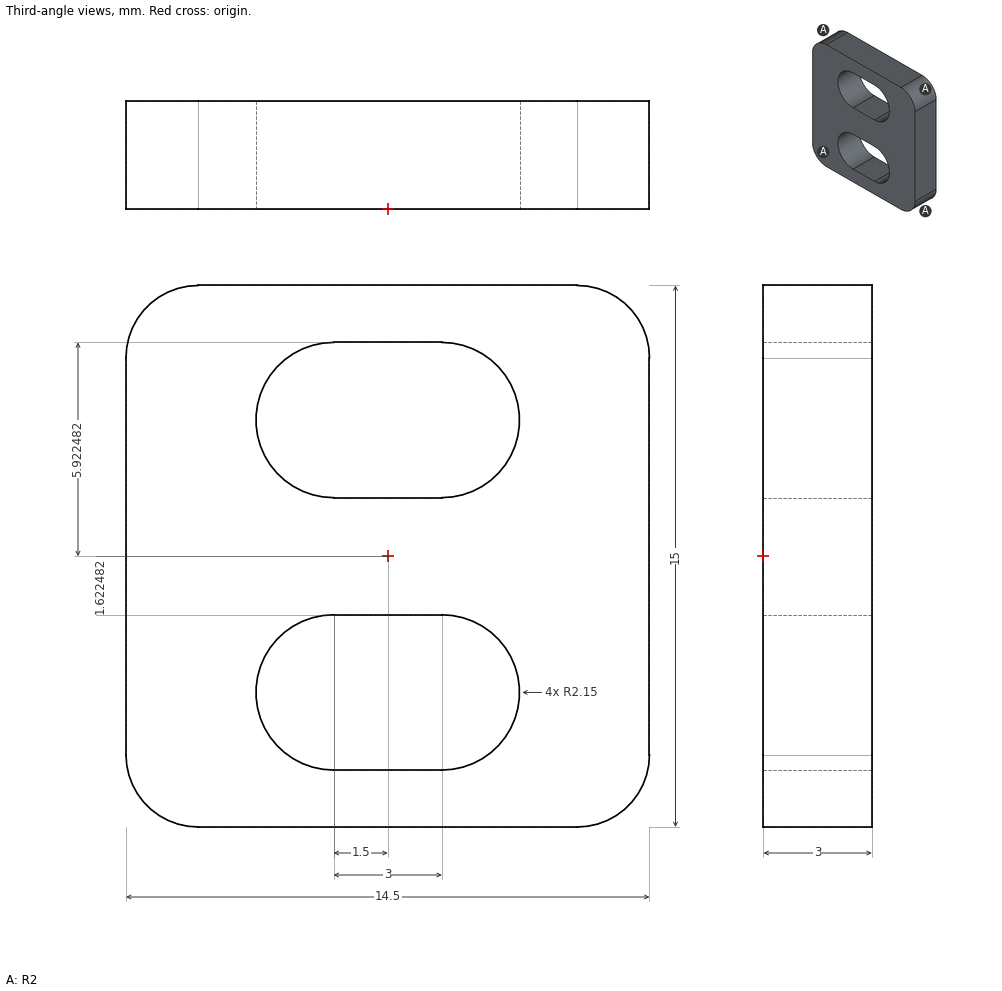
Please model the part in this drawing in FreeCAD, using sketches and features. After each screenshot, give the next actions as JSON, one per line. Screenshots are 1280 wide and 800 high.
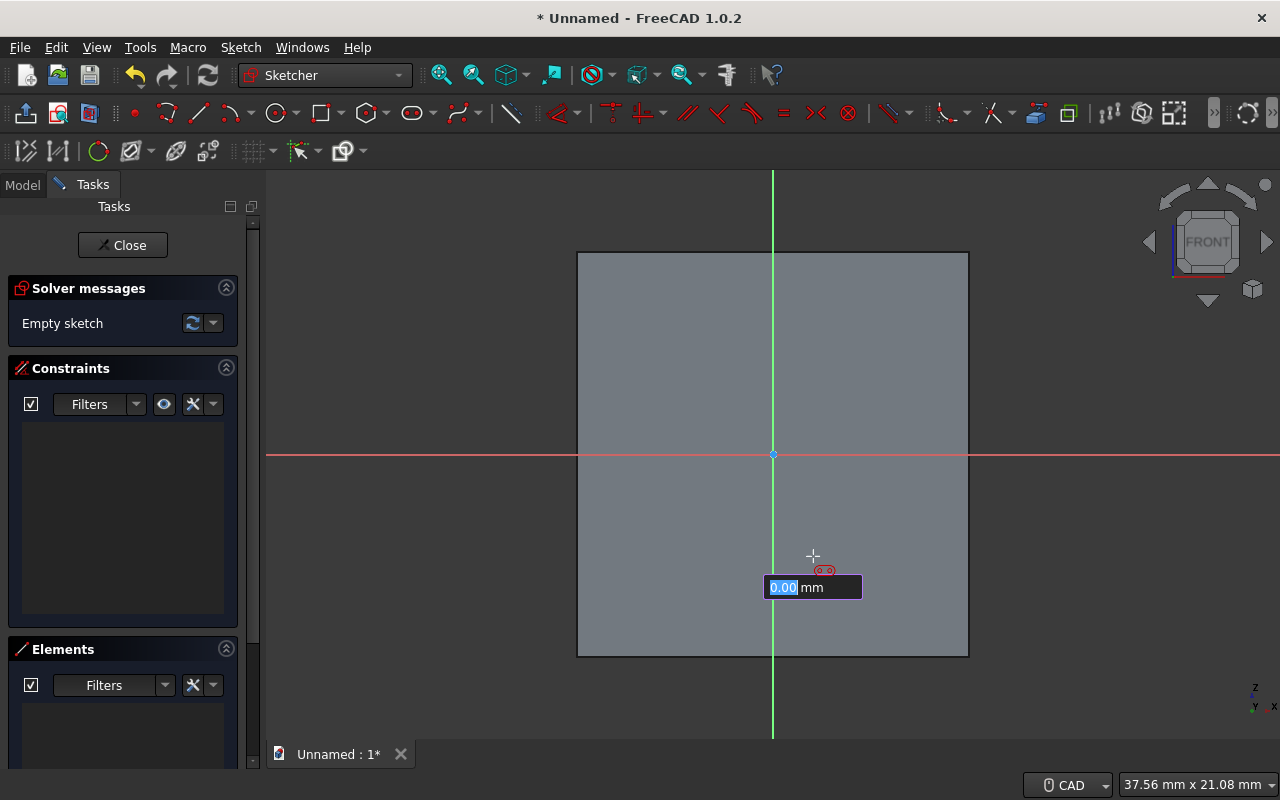
{"action": "scroll", "coordinate": [761, 614], "scroll_direction": "up", "scroll_amount": 2}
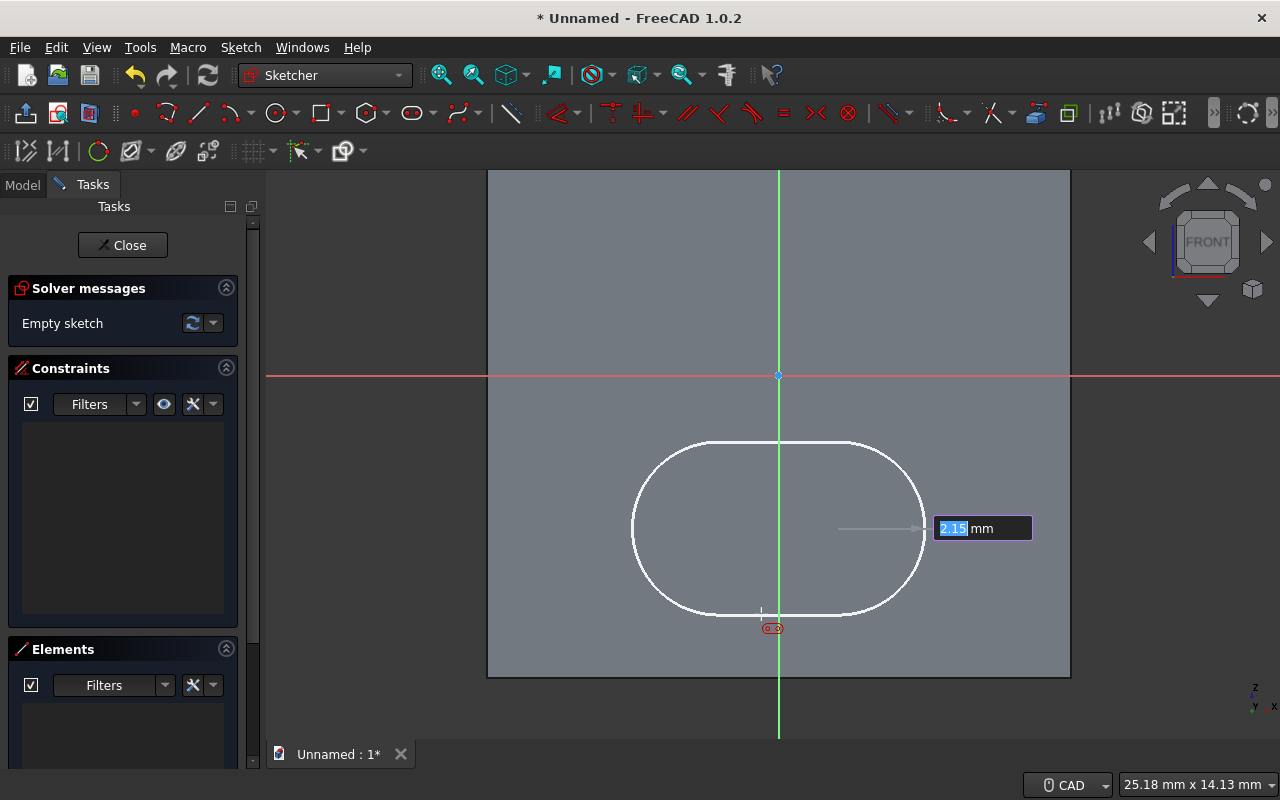
{"action": "left_click", "coordinate": [761, 614]}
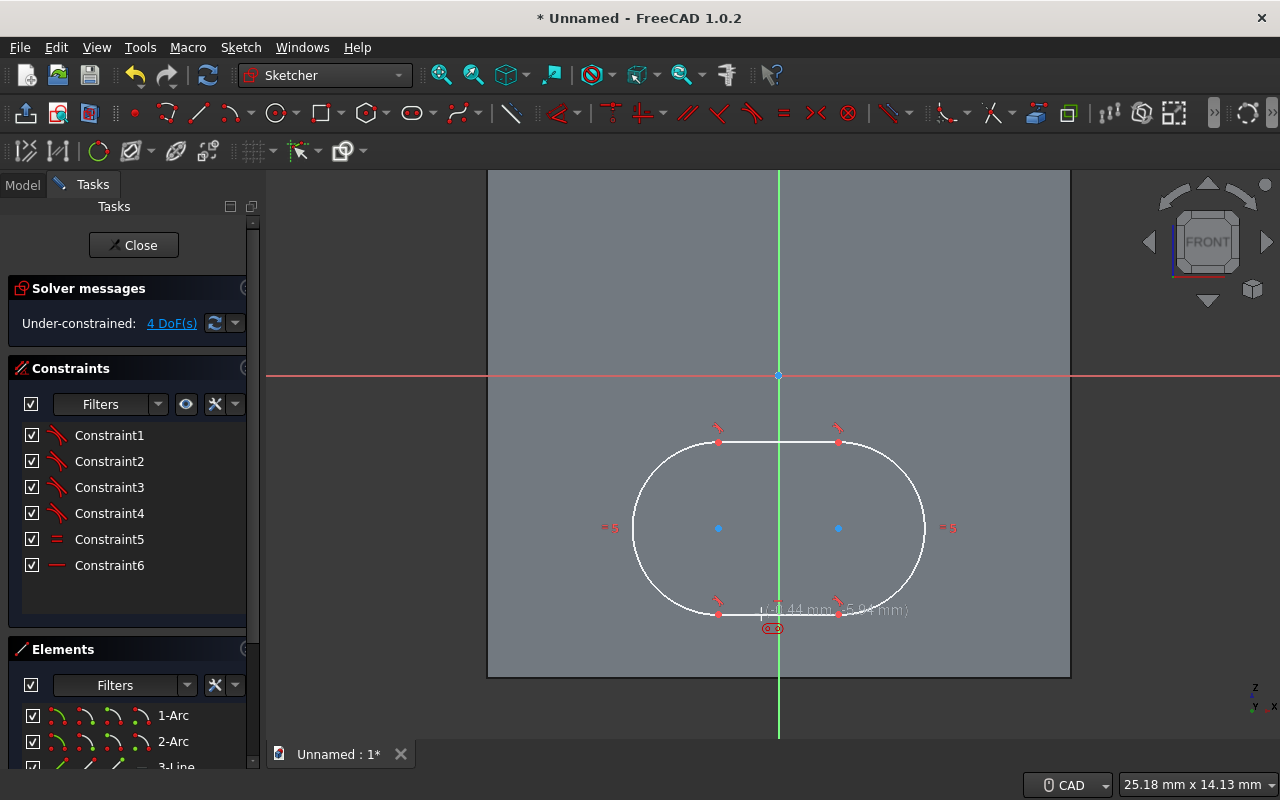
{"action": "left_click", "coordinate": [718, 224]}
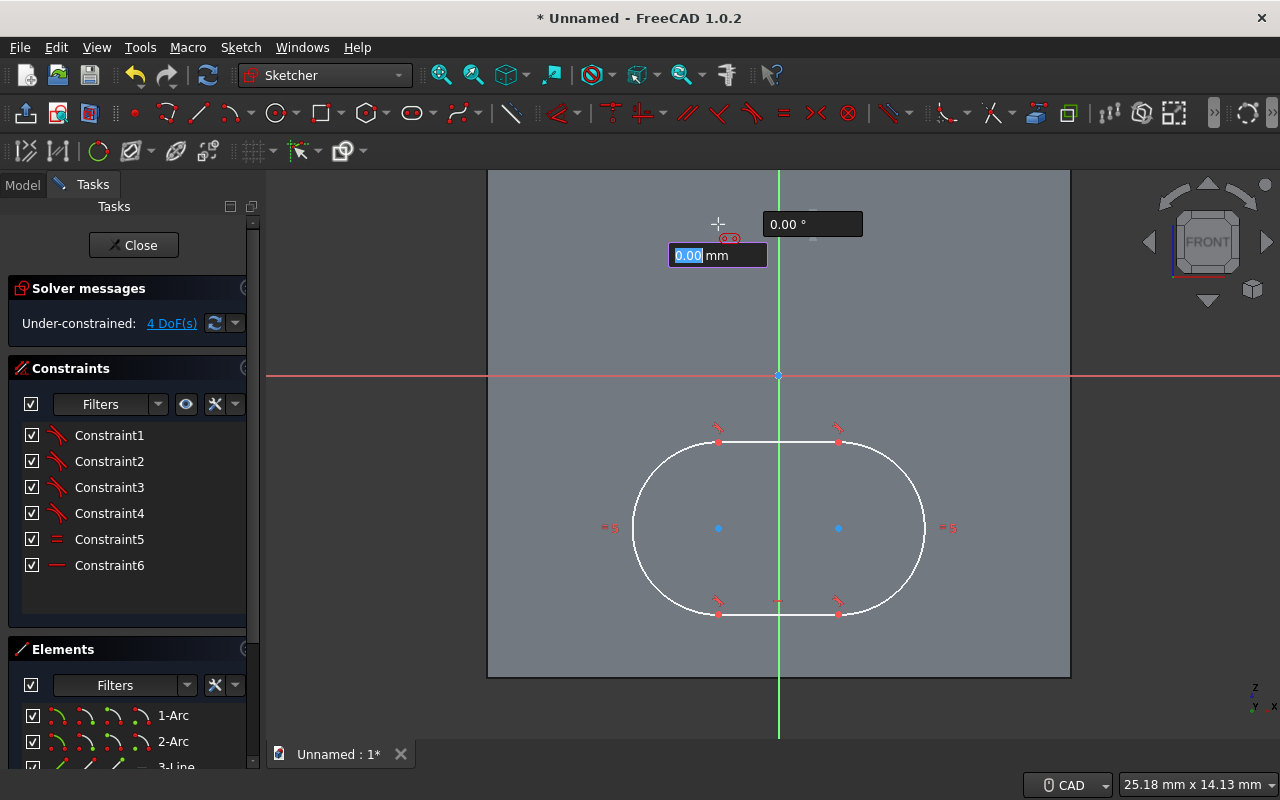
{"action": "left_click", "coordinate": [839, 224]}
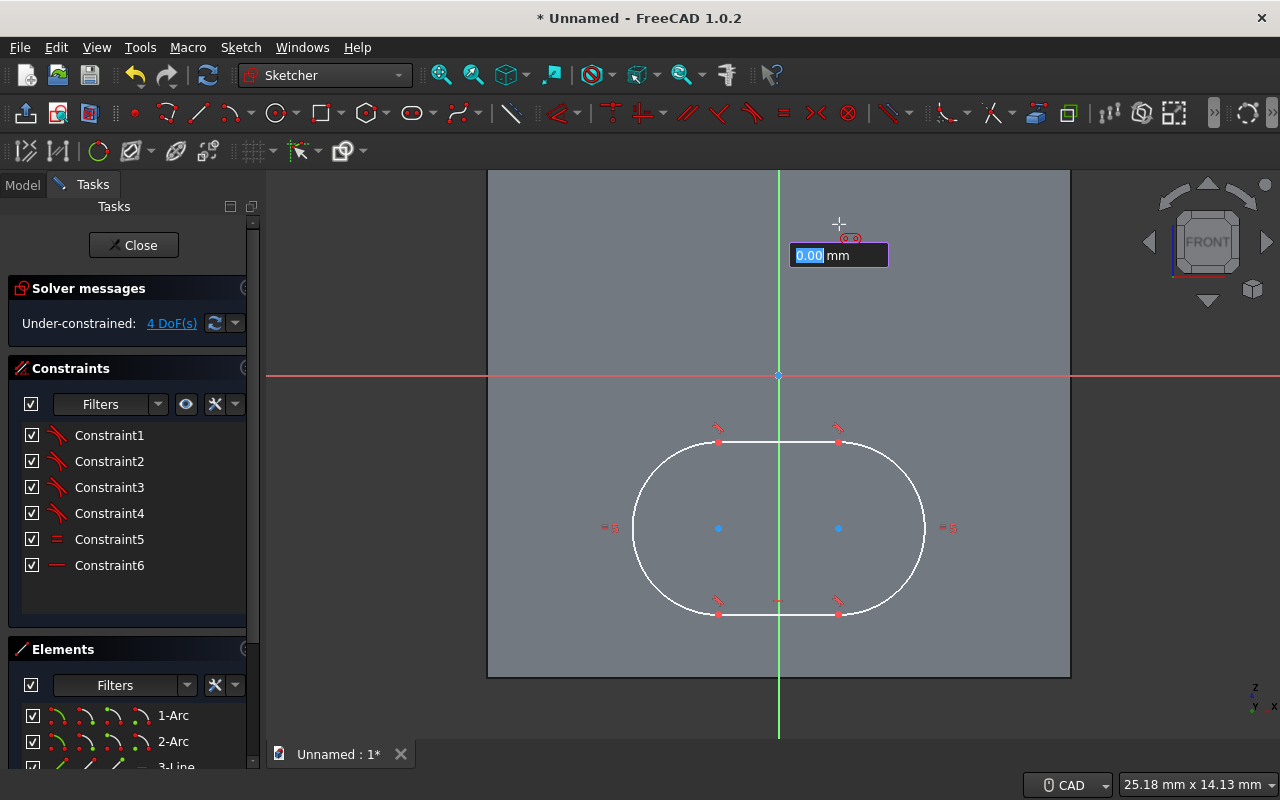
{"action": "scroll", "coordinate": [370, 711], "scroll_direction": "down", "scroll_amount": 1}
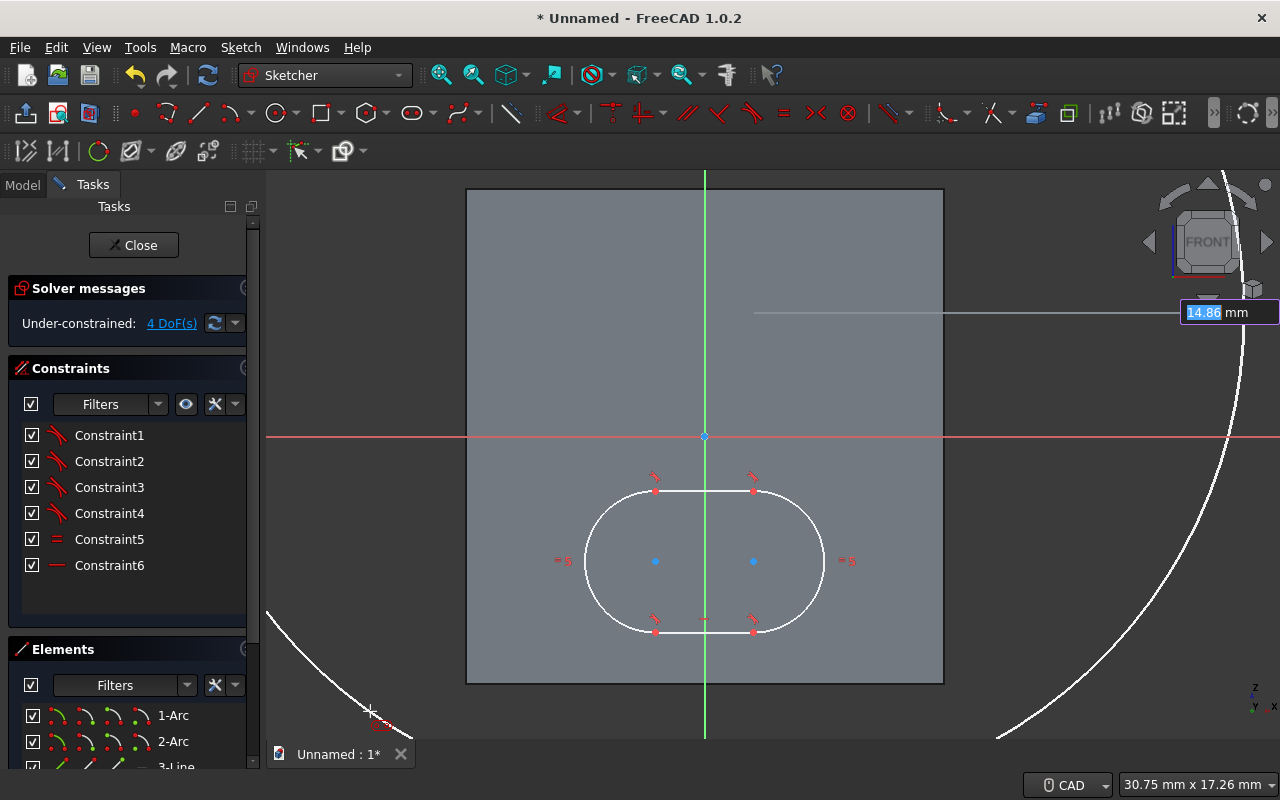
{"action": "left_click", "coordinate": [719, 241]}
{"action": "key", "text": "Escape"}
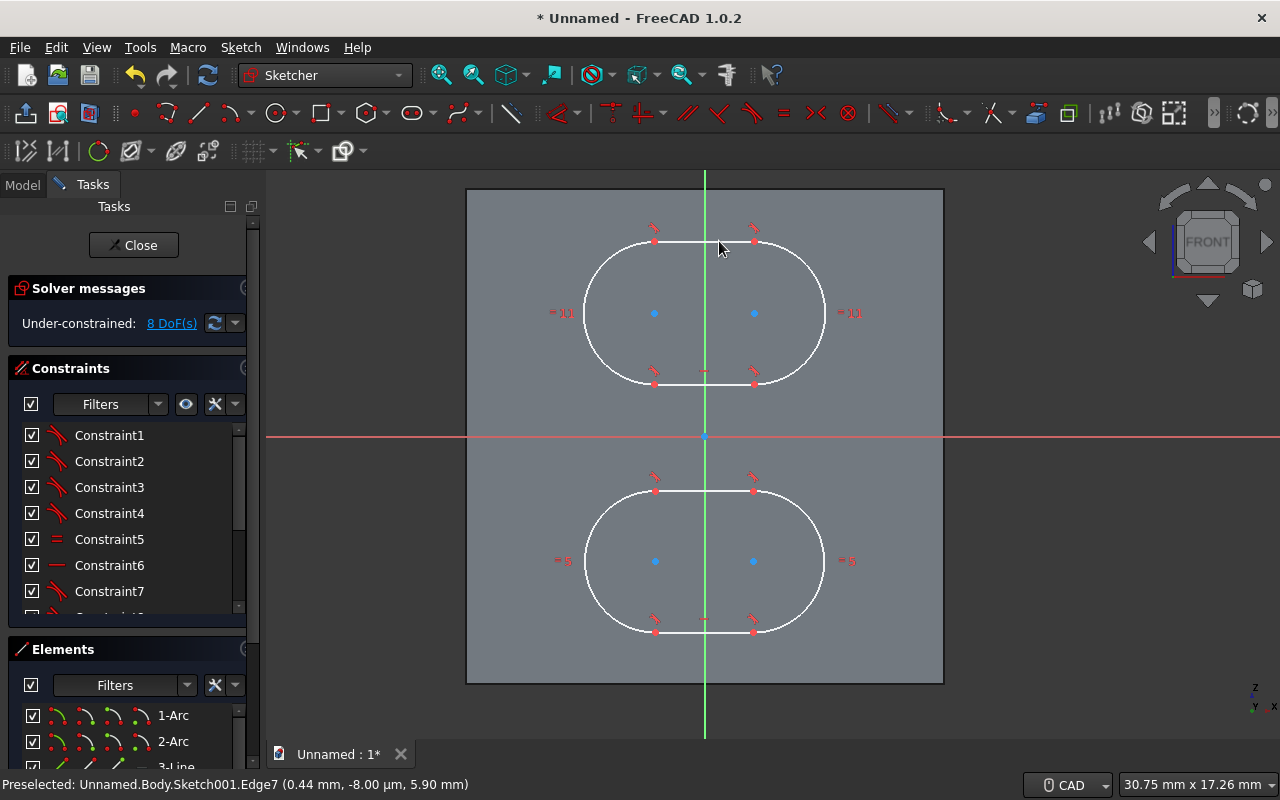
{"action": "left_click", "coordinate": [599, 520]}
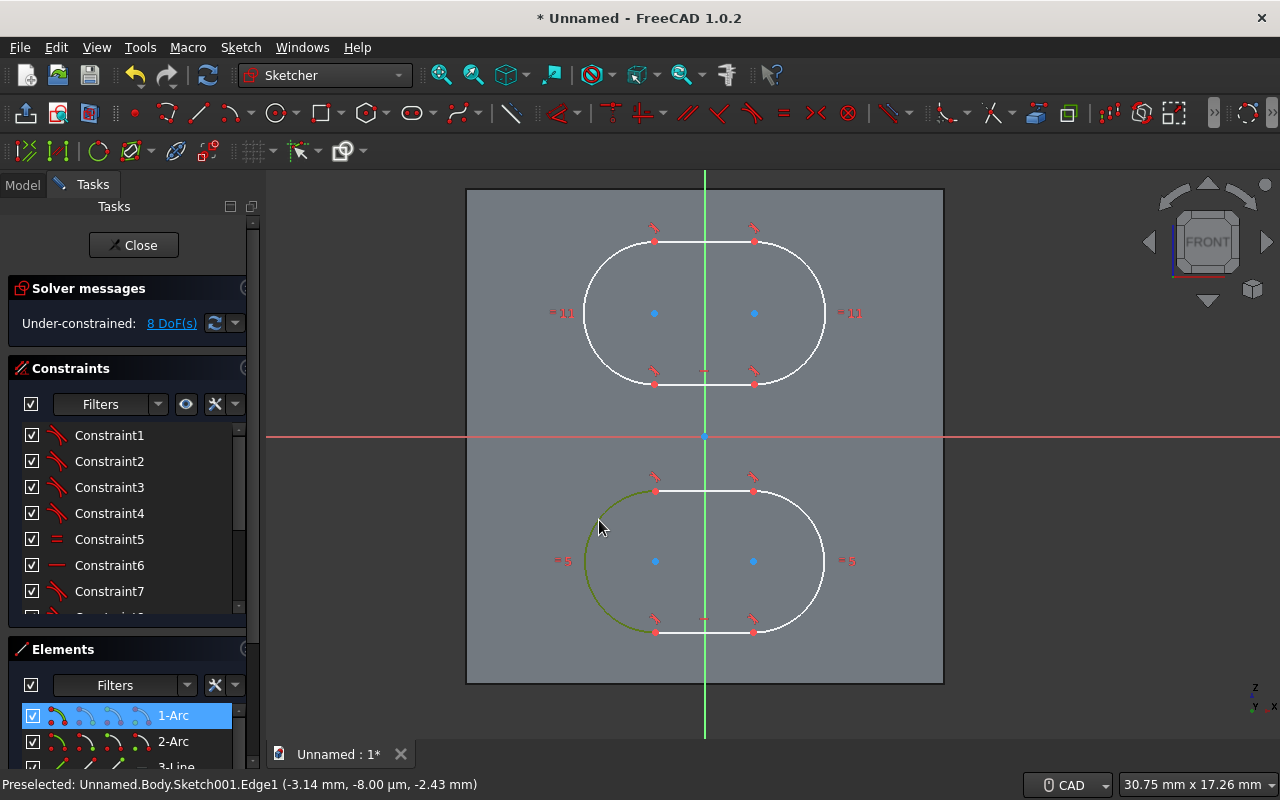
{"action": "left_click", "coordinate": [597, 271]}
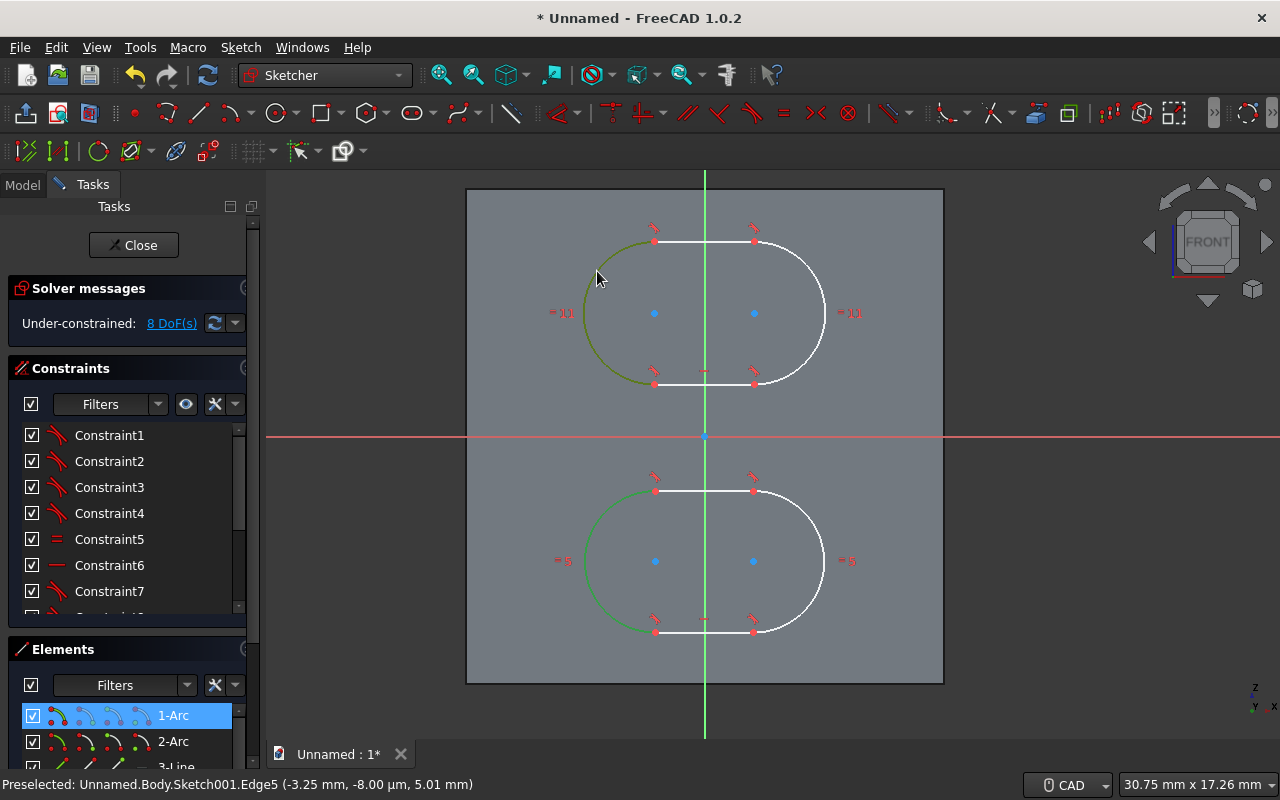
{"action": "left_click", "coordinate": [784, 114]}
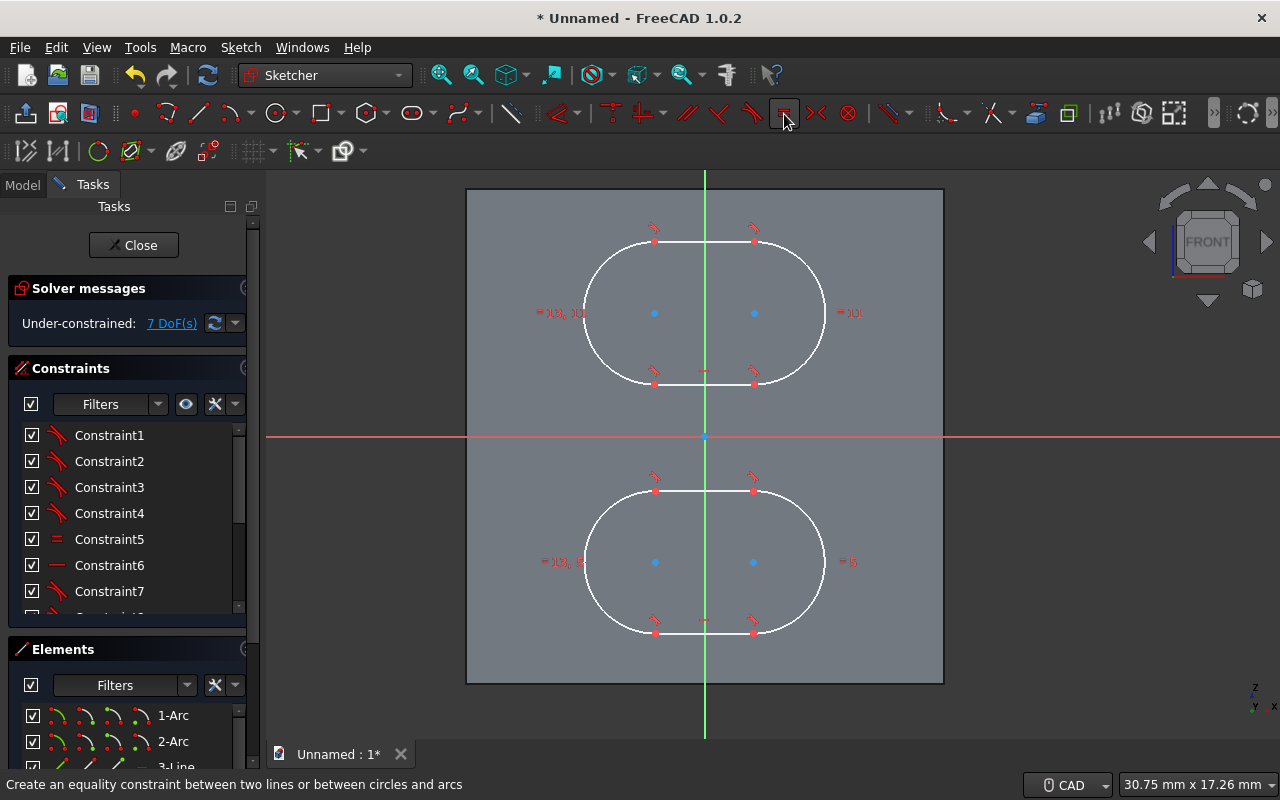
{"action": "left_click", "coordinate": [558, 114]}